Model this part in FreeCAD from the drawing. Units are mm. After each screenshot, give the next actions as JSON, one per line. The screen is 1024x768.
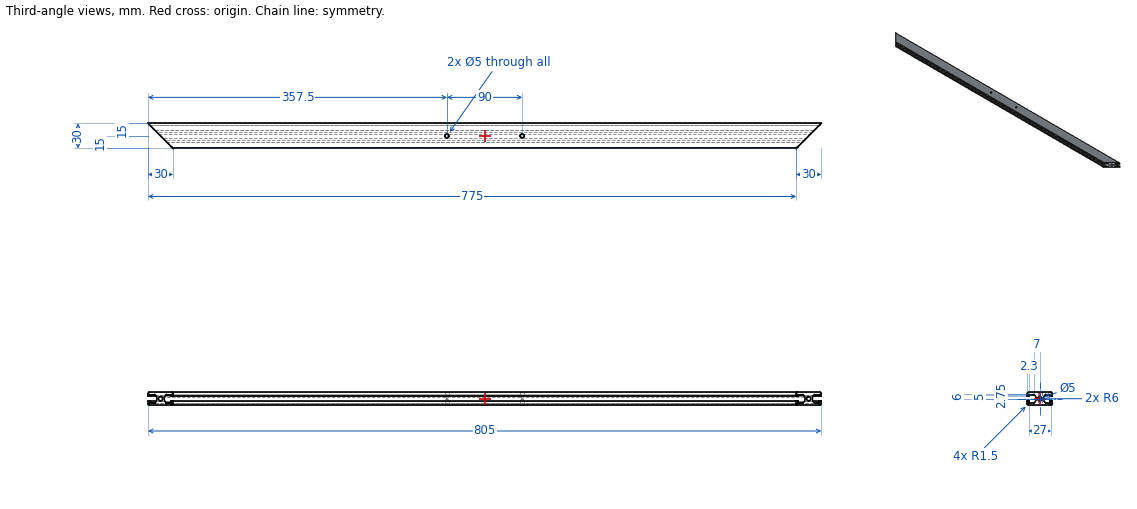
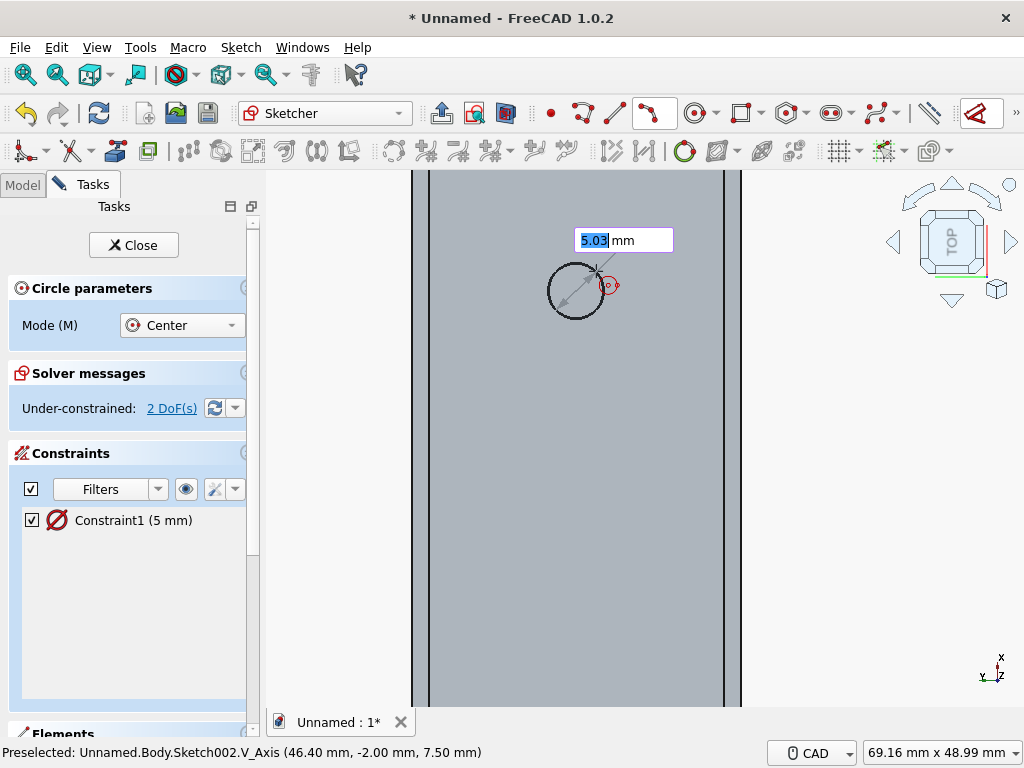
{"action": "type", "text": "5"}
{"action": "key", "text": "Return"}
{"action": "key", "text": "Escape"}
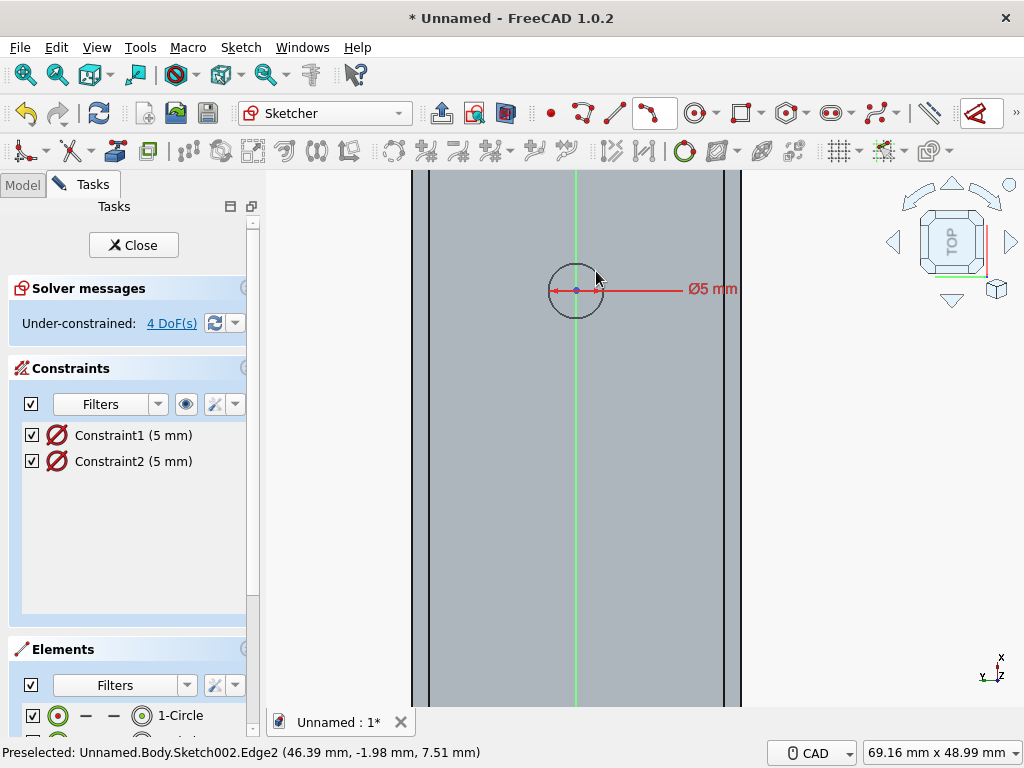
{"action": "scroll", "coordinate": [577, 290], "scroll_direction": "down", "scroll_amount": 6}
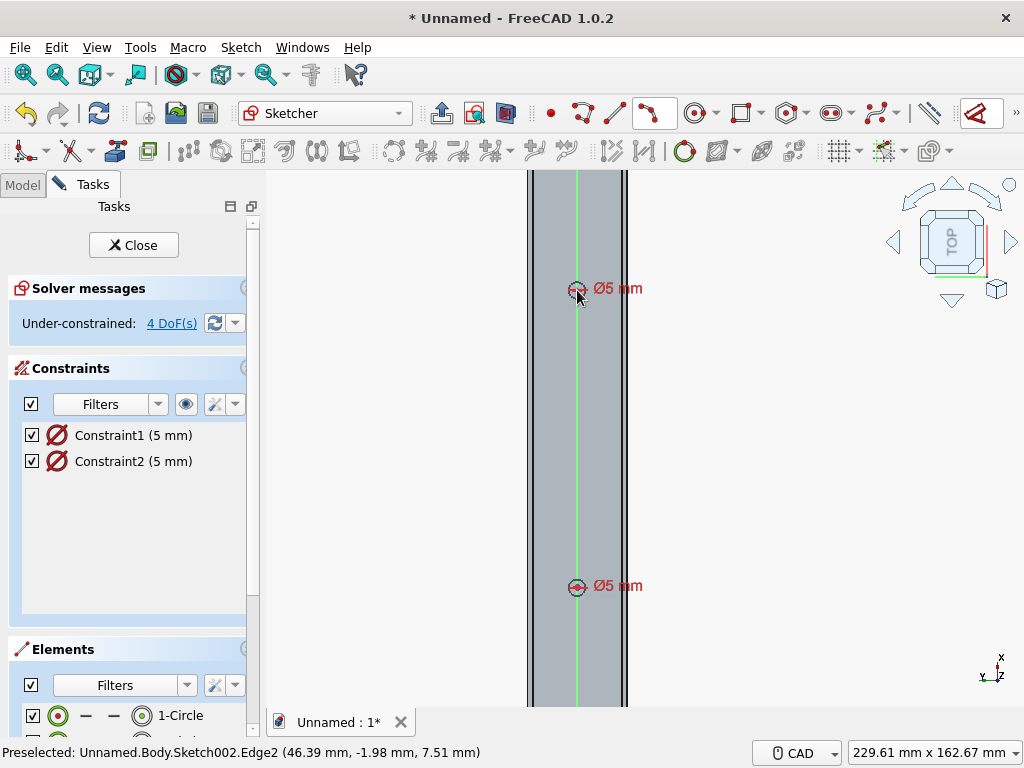
{"action": "left_click", "coordinate": [577, 588]}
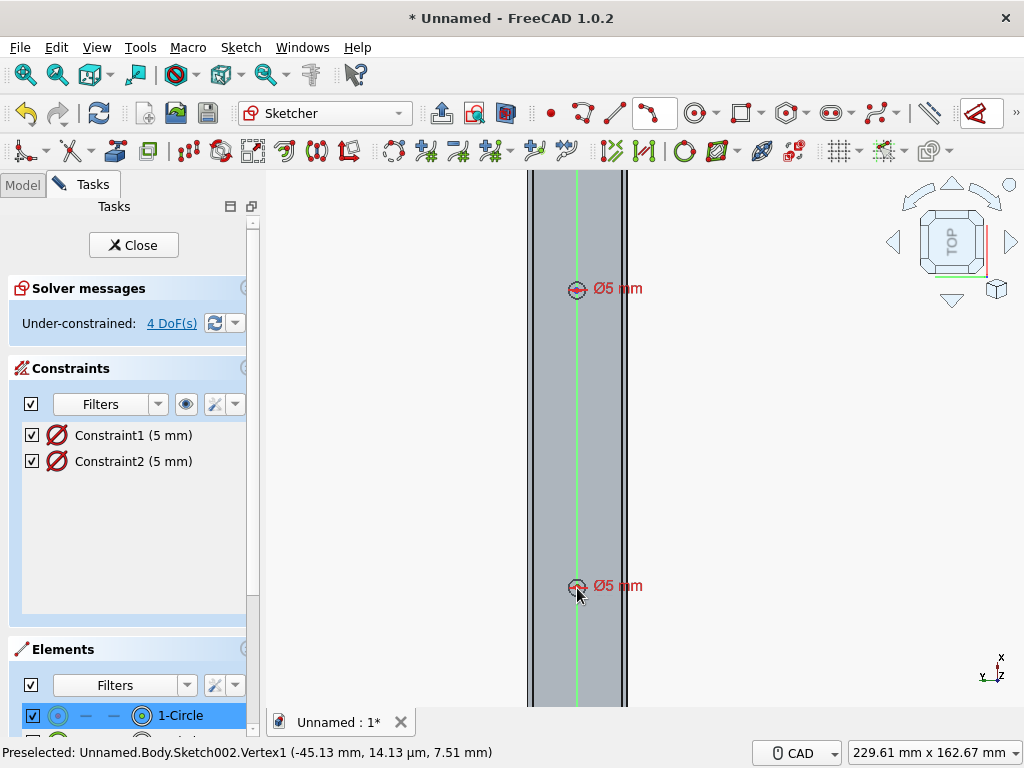
{"action": "left_click", "coordinate": [577, 645]}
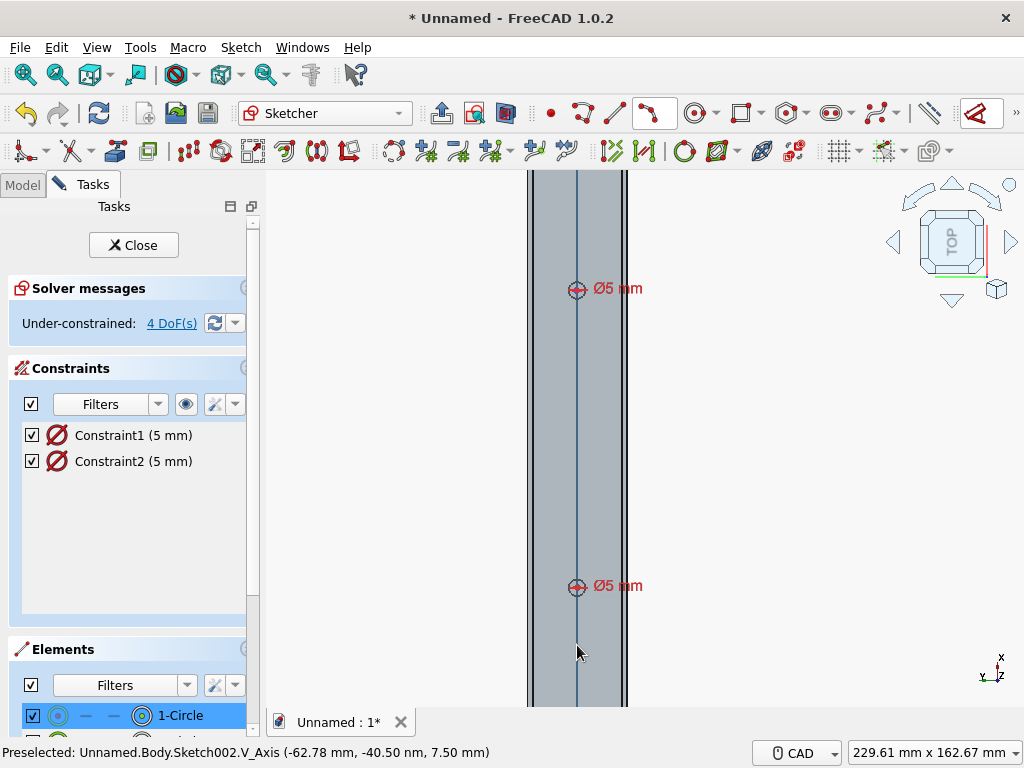
{"action": "key", "text": "c"}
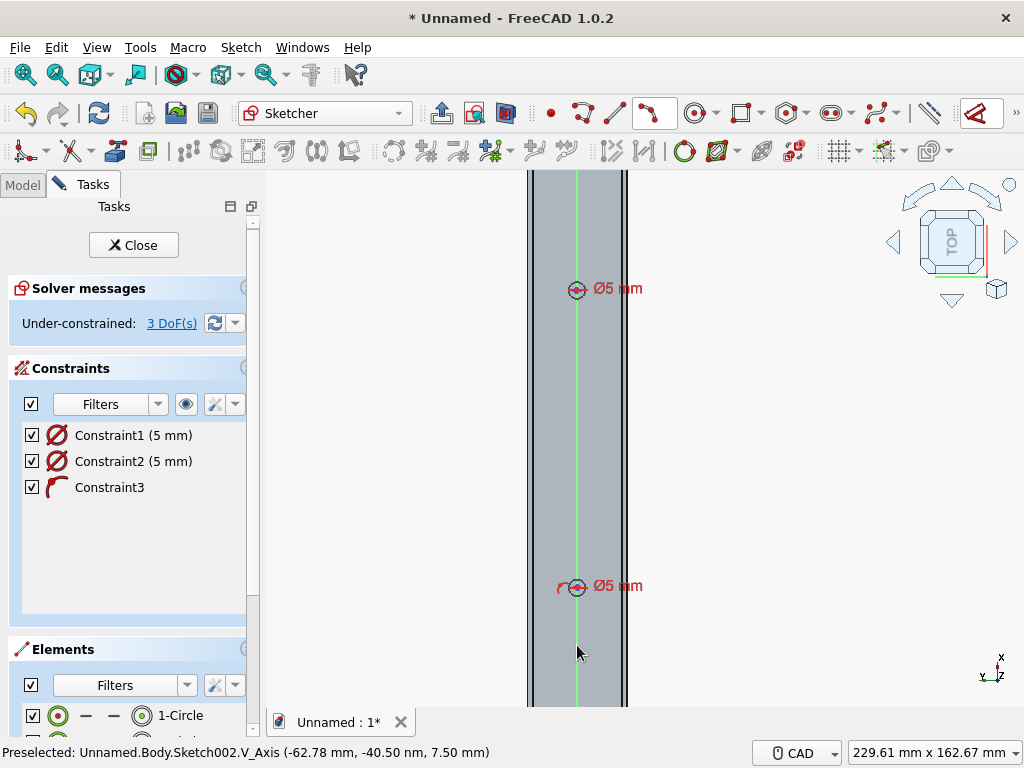
{"action": "left_click", "coordinate": [577, 290]}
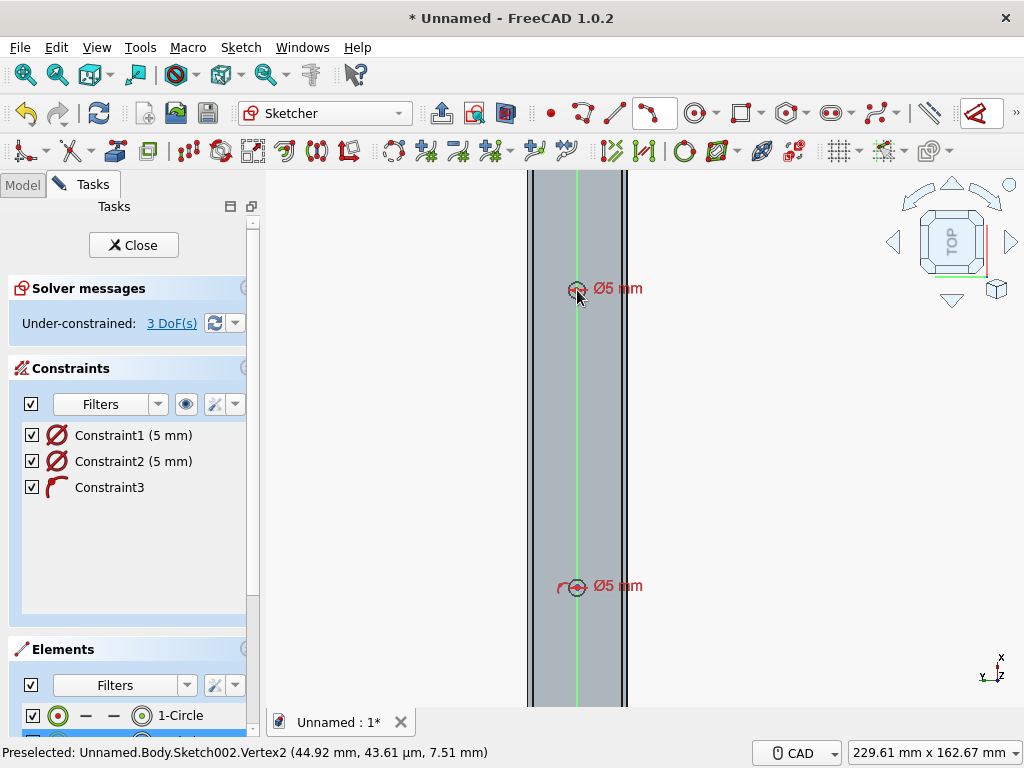
{"action": "left_click", "coordinate": [577, 645]}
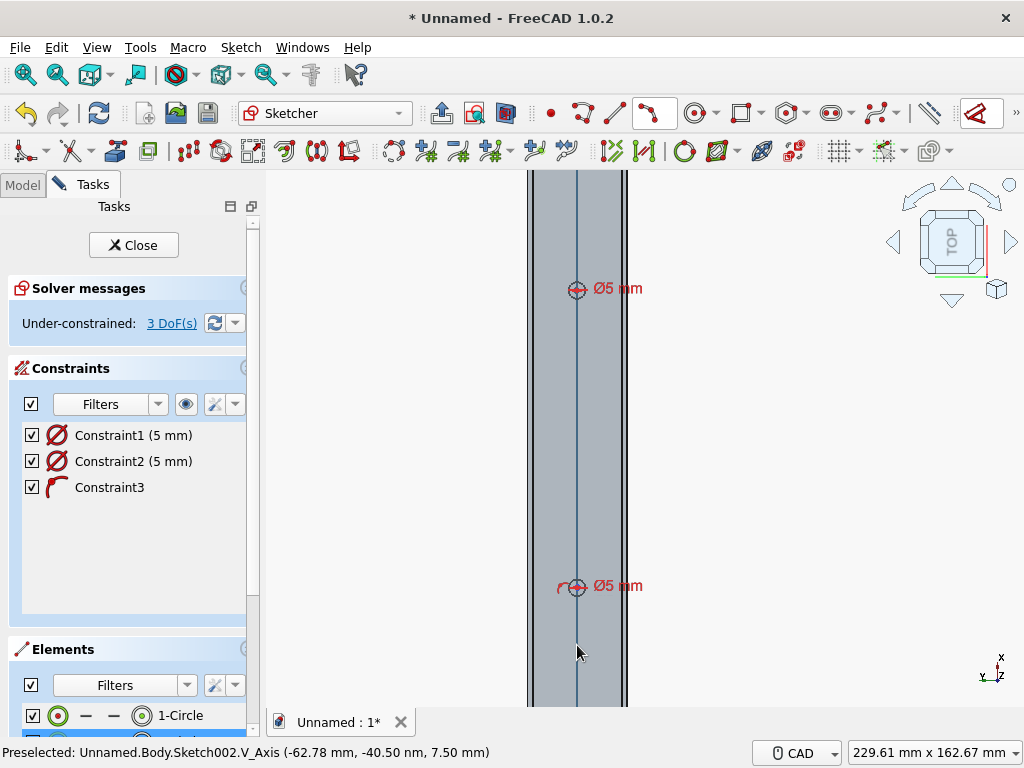
{"action": "key", "text": "c"}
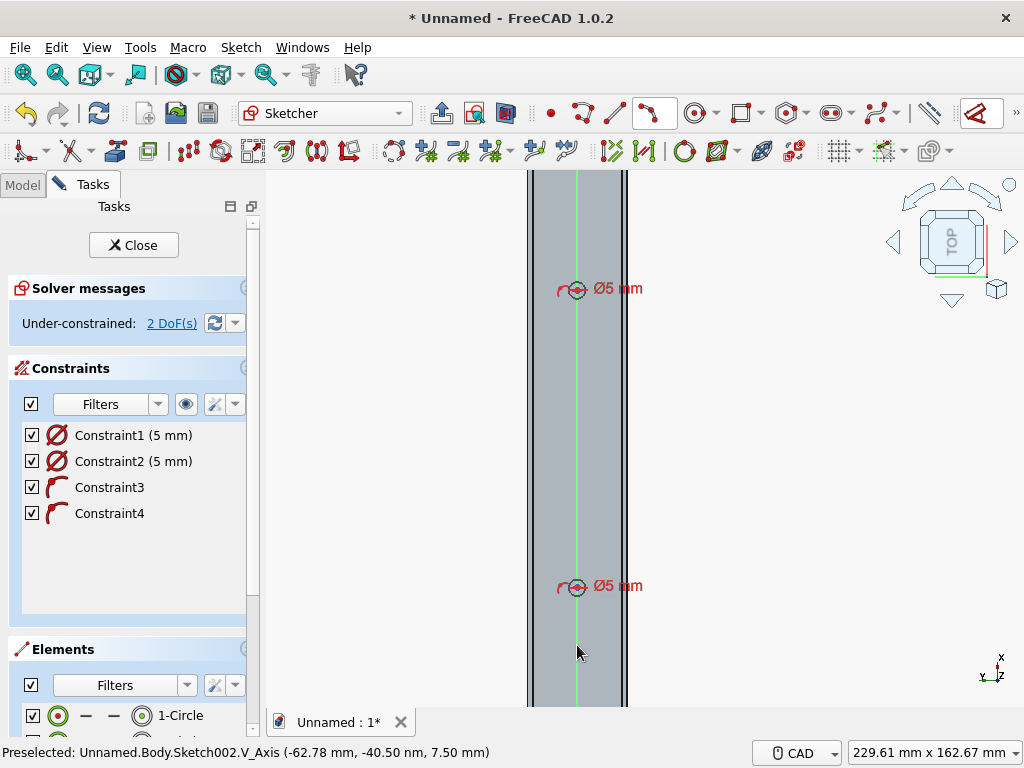
{"action": "left_click", "coordinate": [577, 588]}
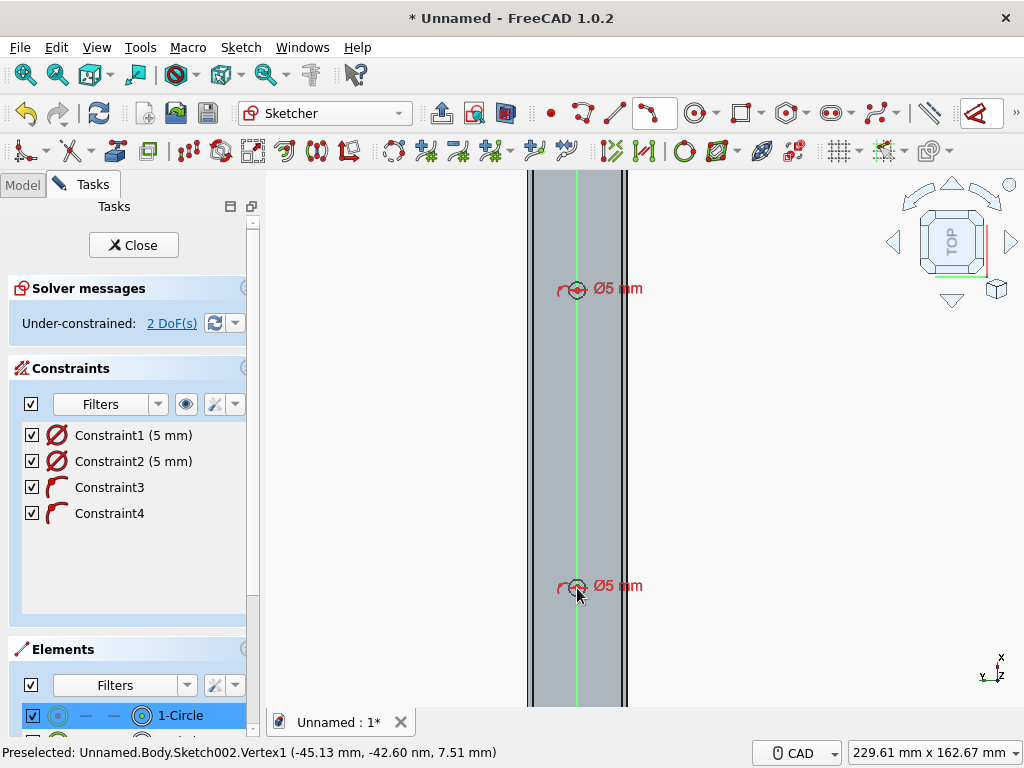
{"action": "left_click", "coordinate": [577, 290]}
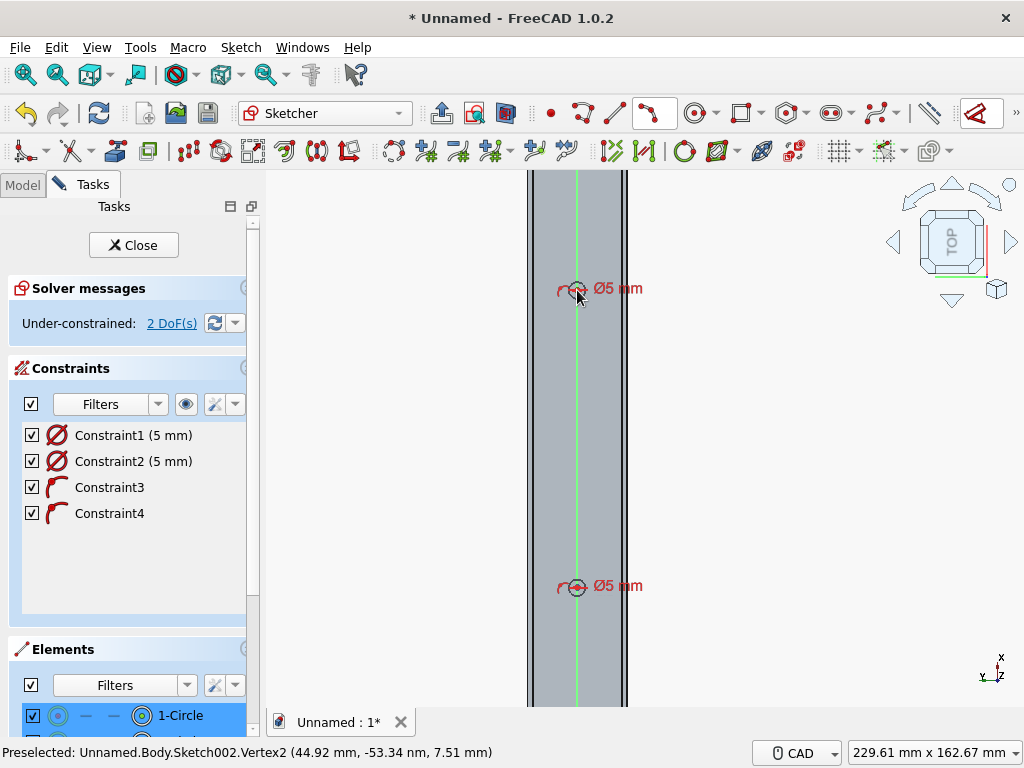
{"action": "key", "text": "i"}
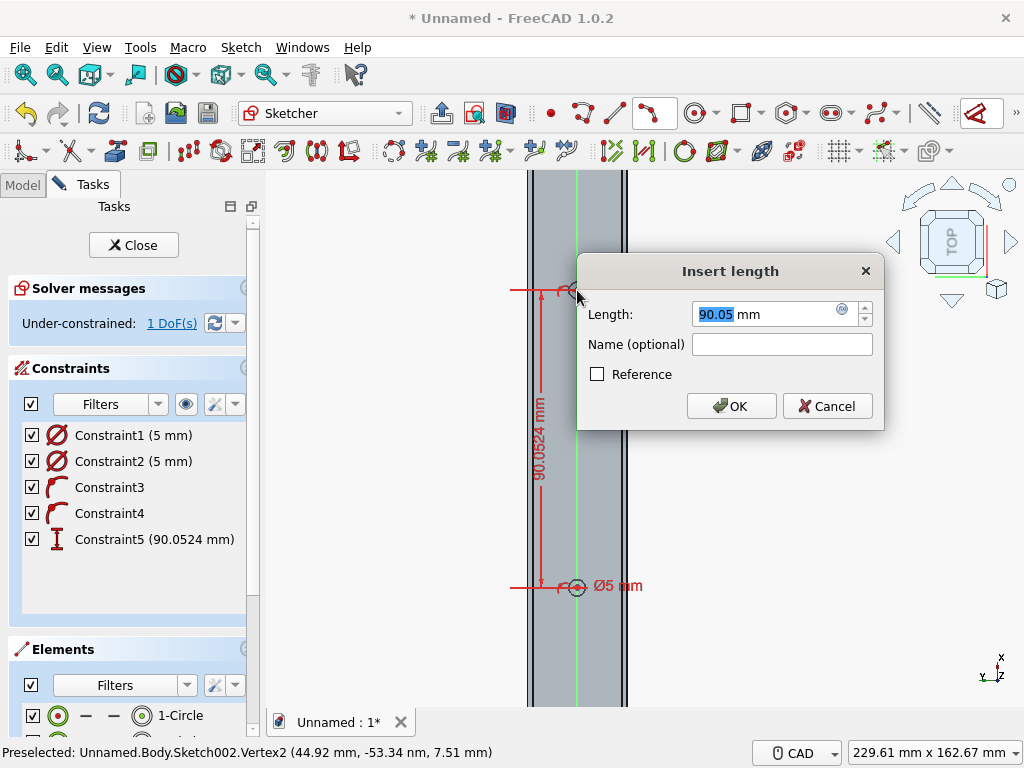
{"action": "type", "text": "90"}
{"action": "key", "text": "Return"}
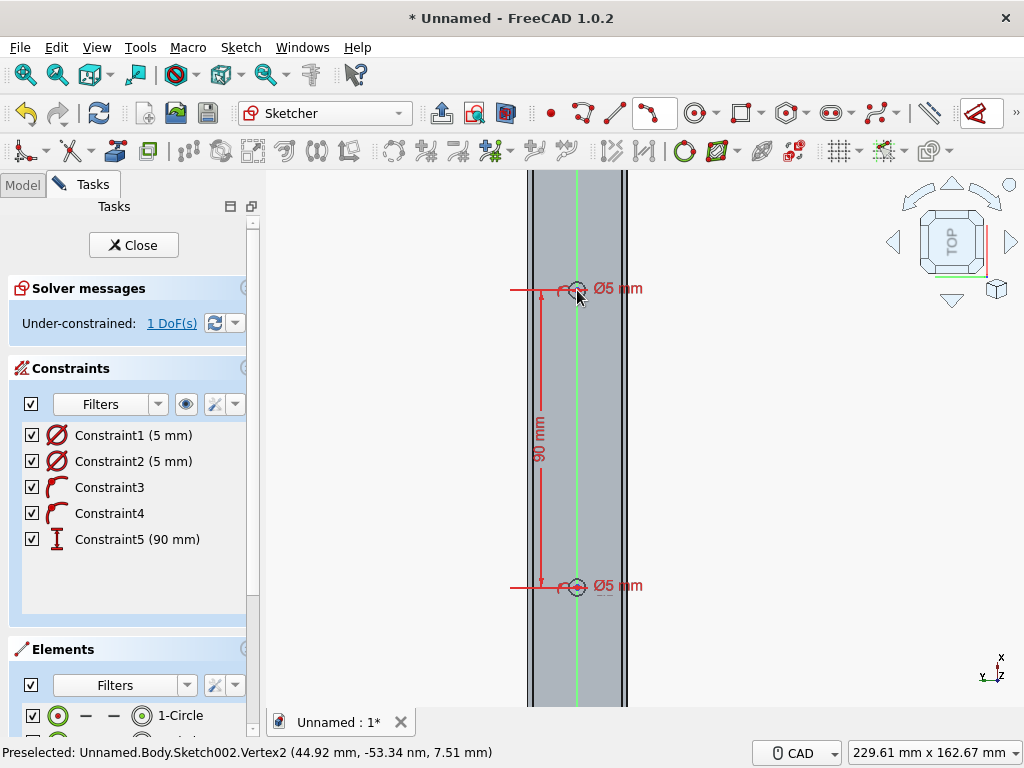
{"action": "left_click", "coordinate": [577, 588]}